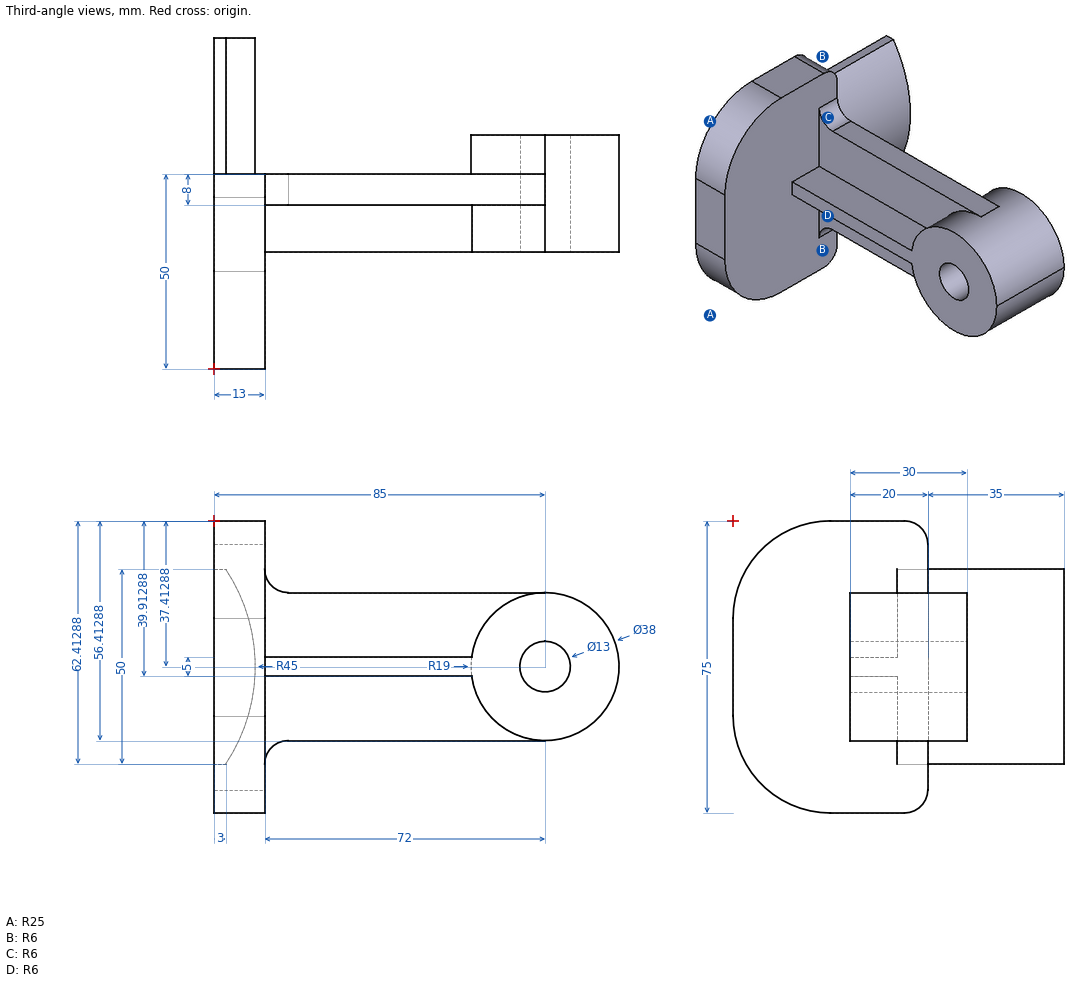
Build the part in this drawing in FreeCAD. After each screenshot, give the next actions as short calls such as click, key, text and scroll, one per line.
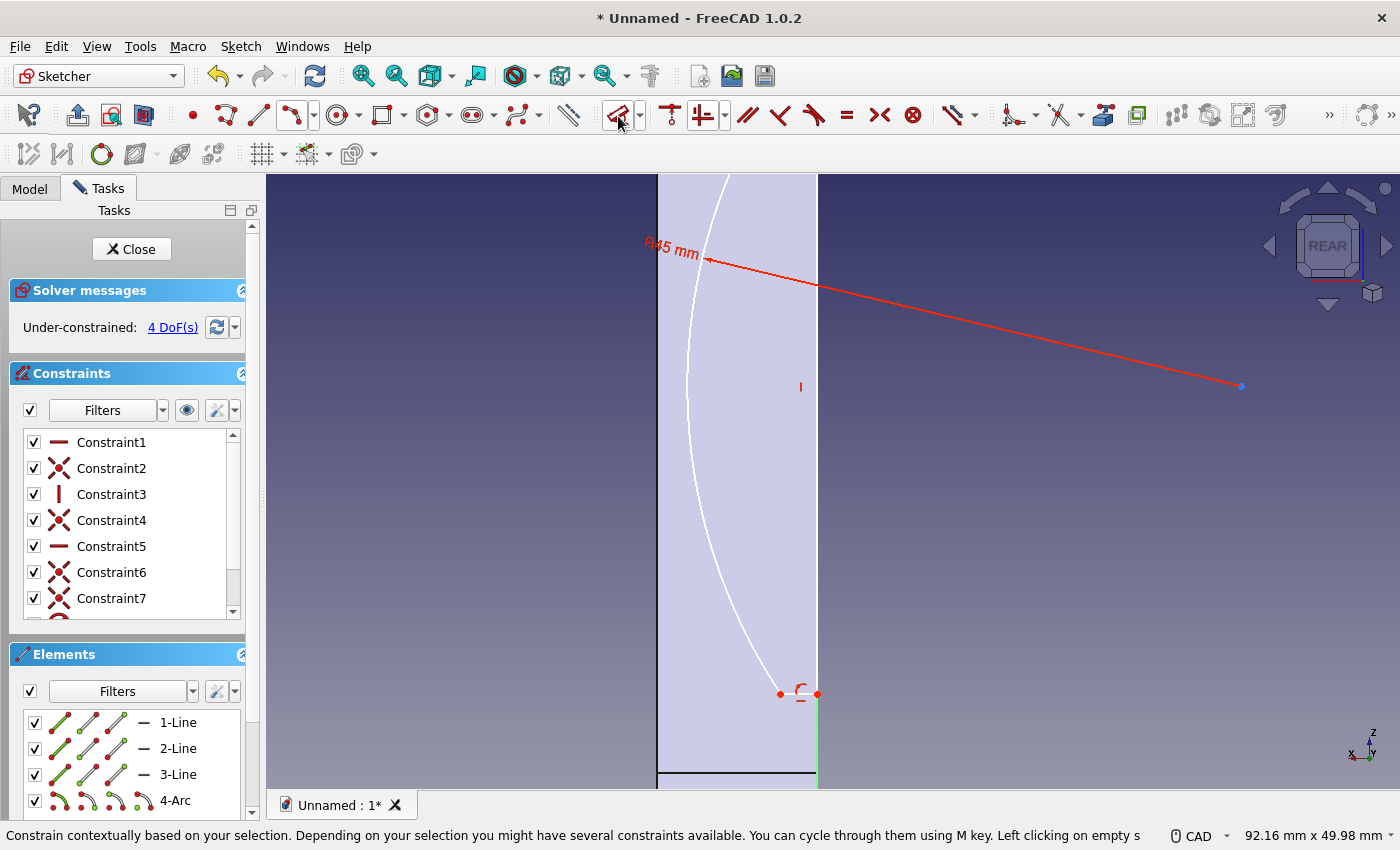
scroll(792, 694, up, 2)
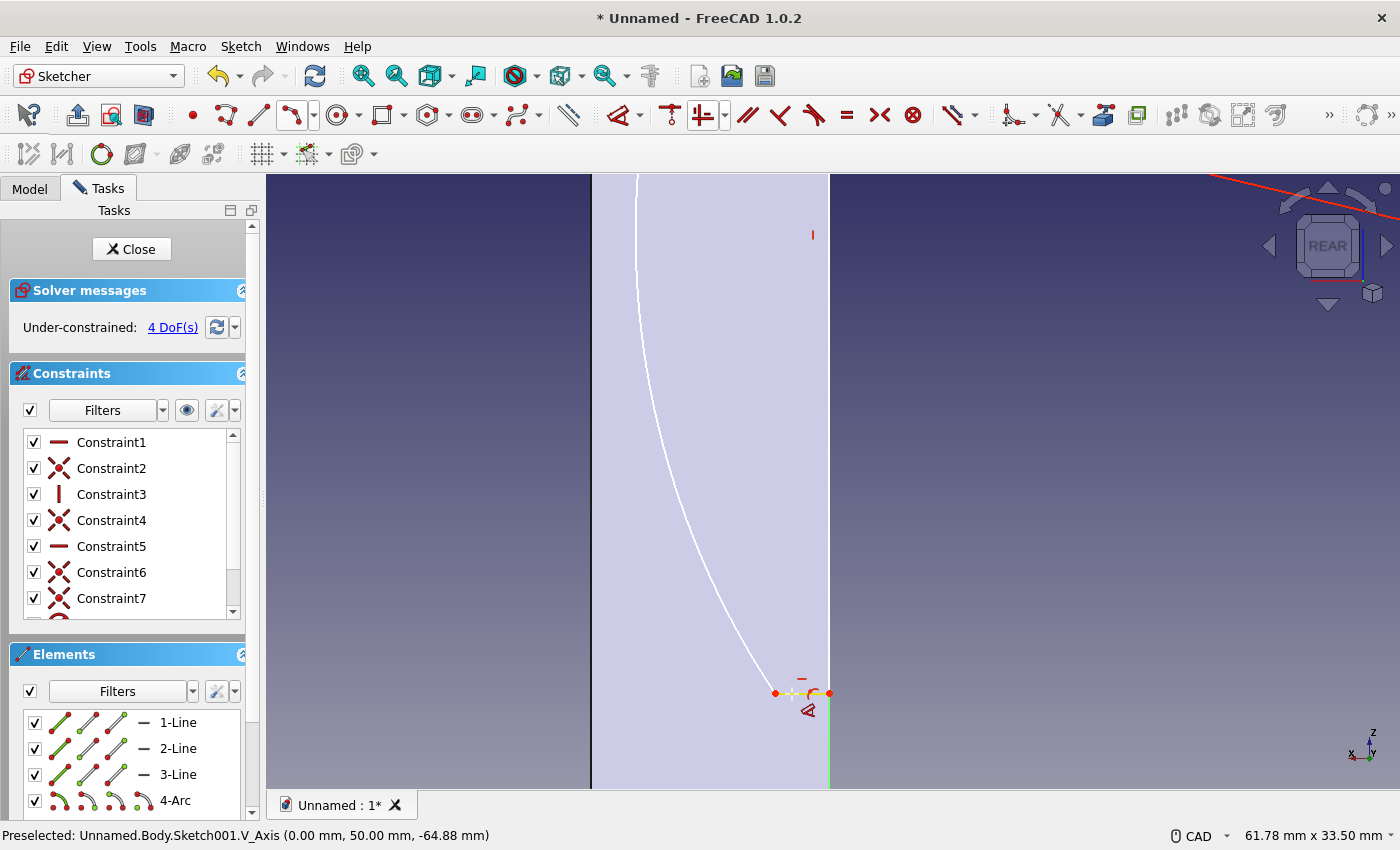
click(791, 694)
click(802, 728)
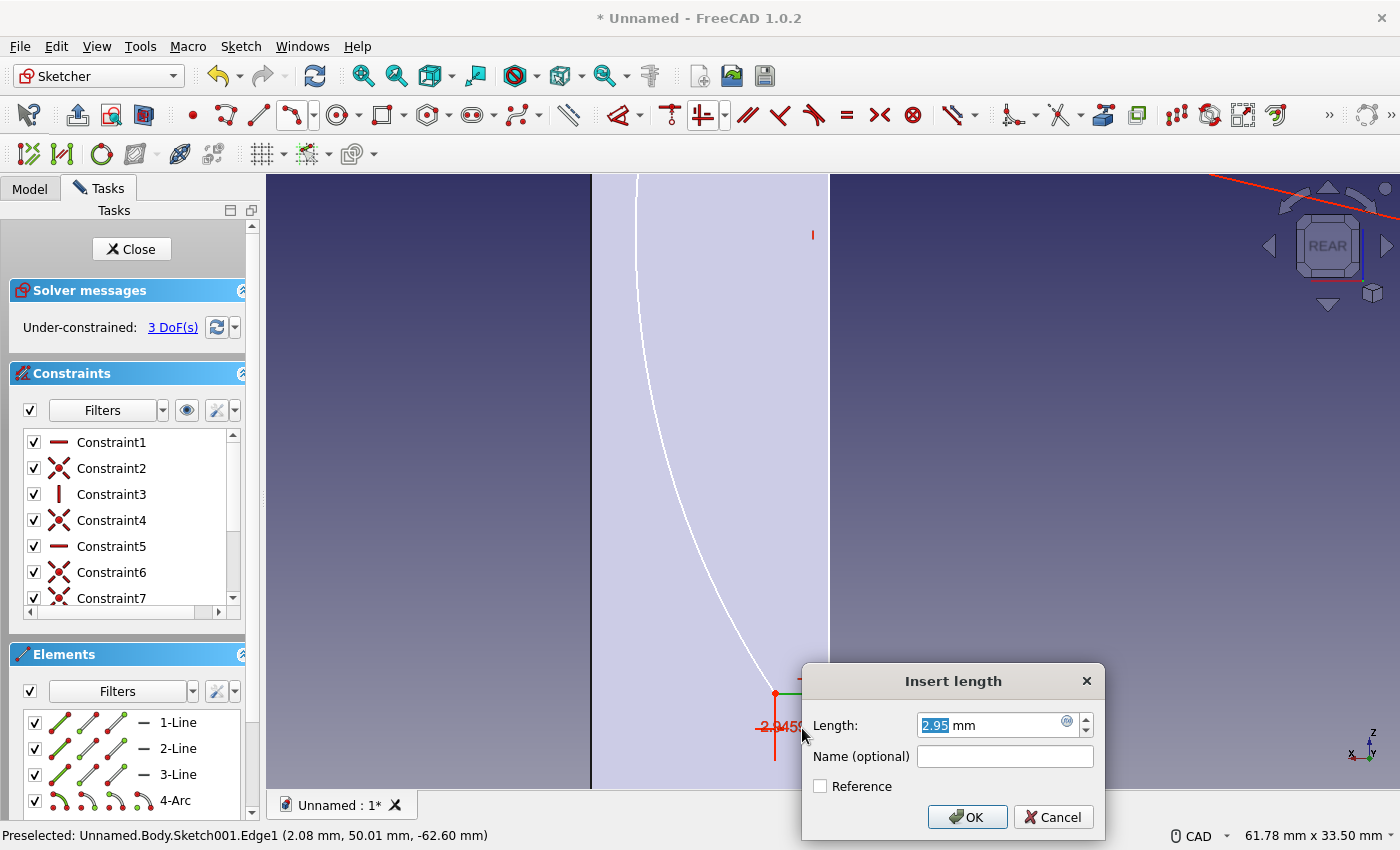
text(3)
key(Return)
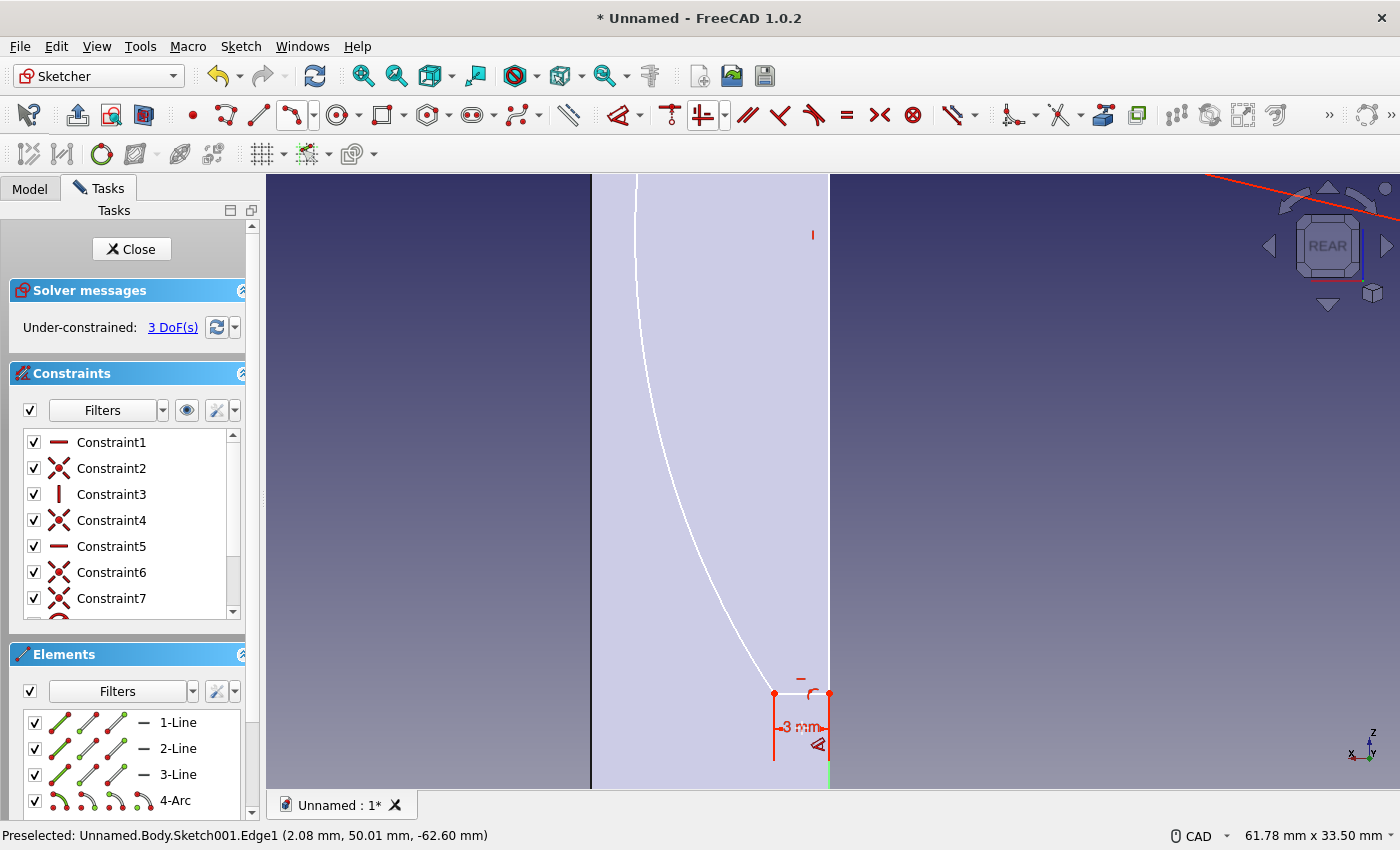
scroll(783, 693, down, 5)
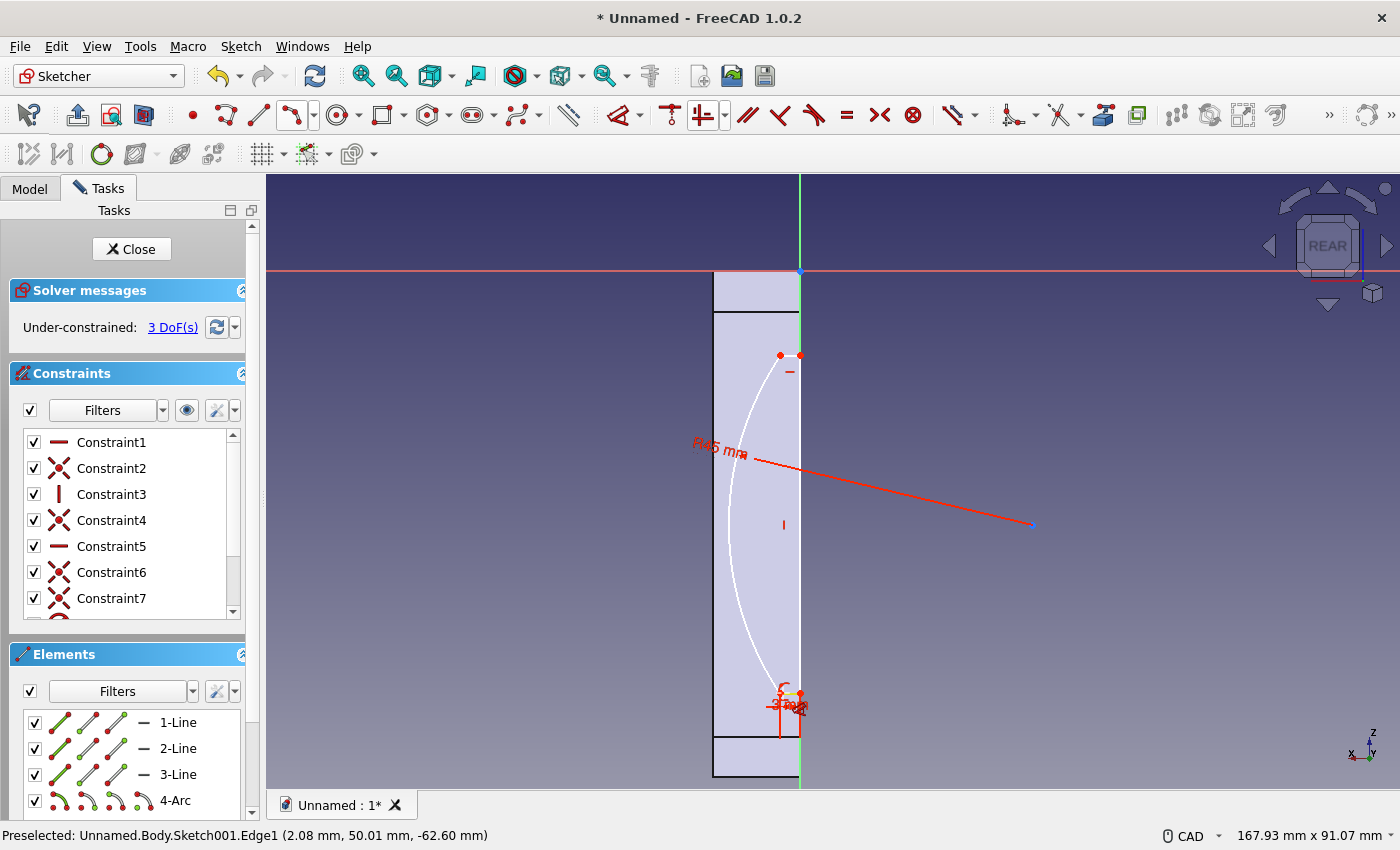
scroll(794, 356, up, 5)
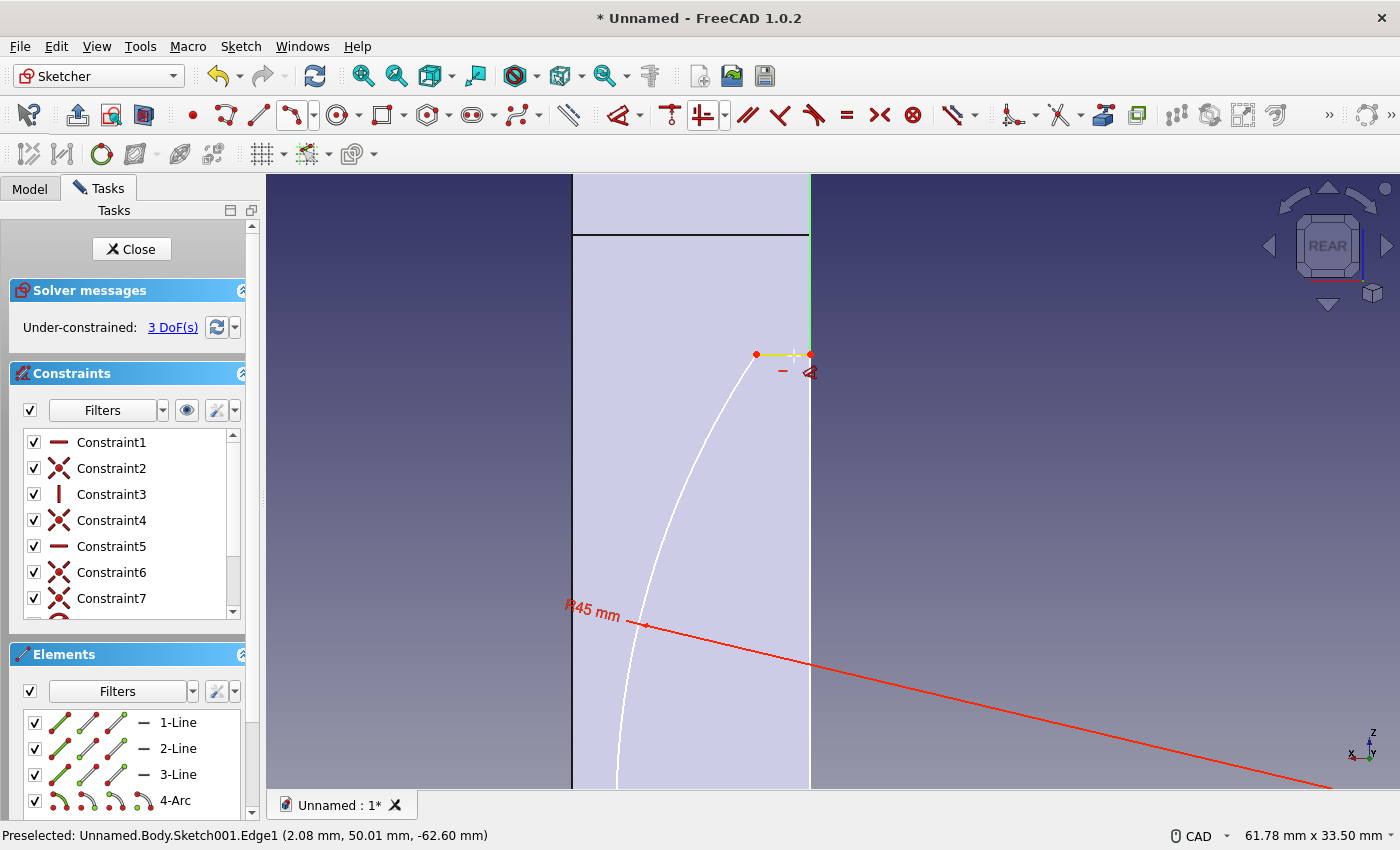
click(794, 355)
click(783, 321)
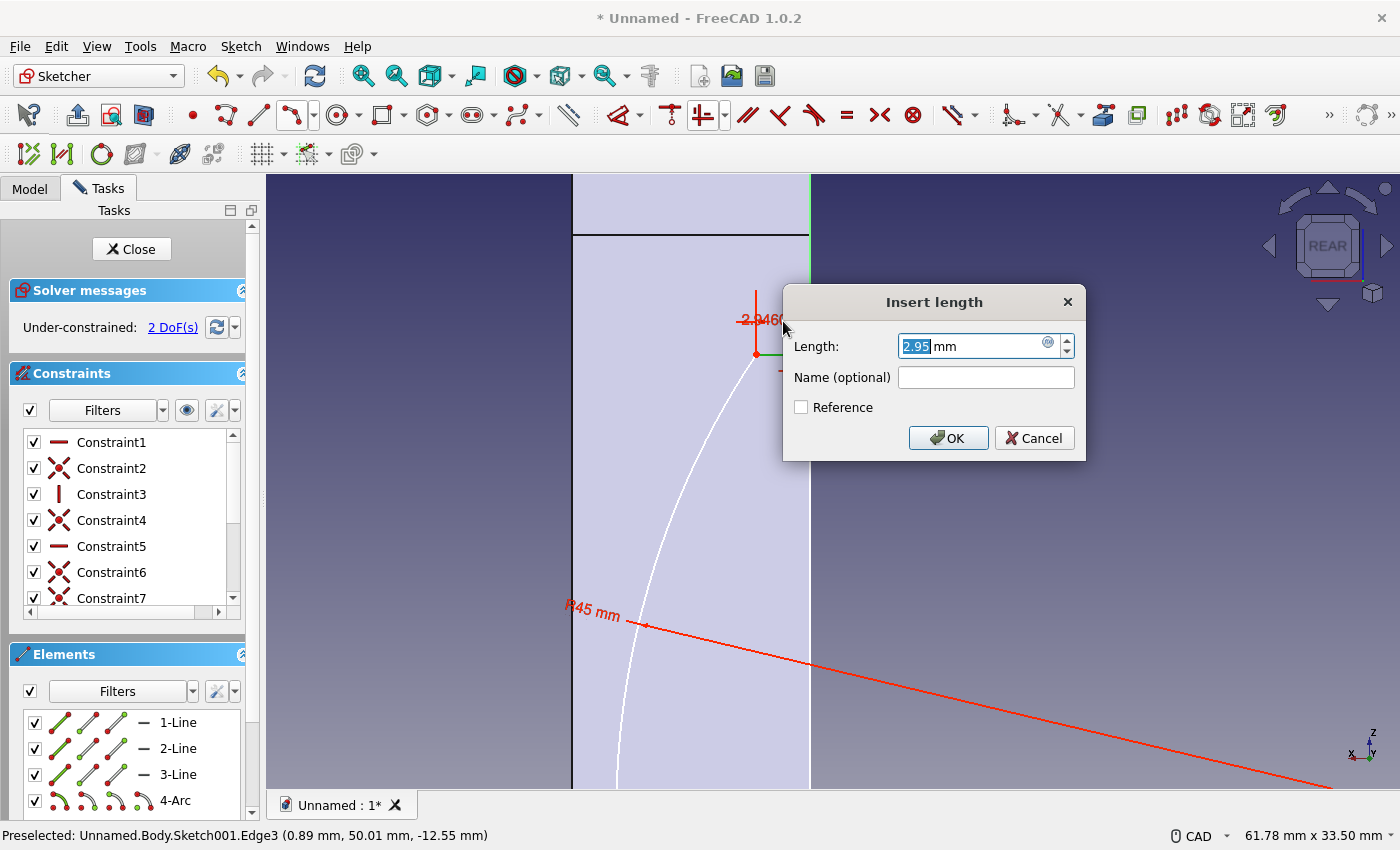
text(3)
key(Return)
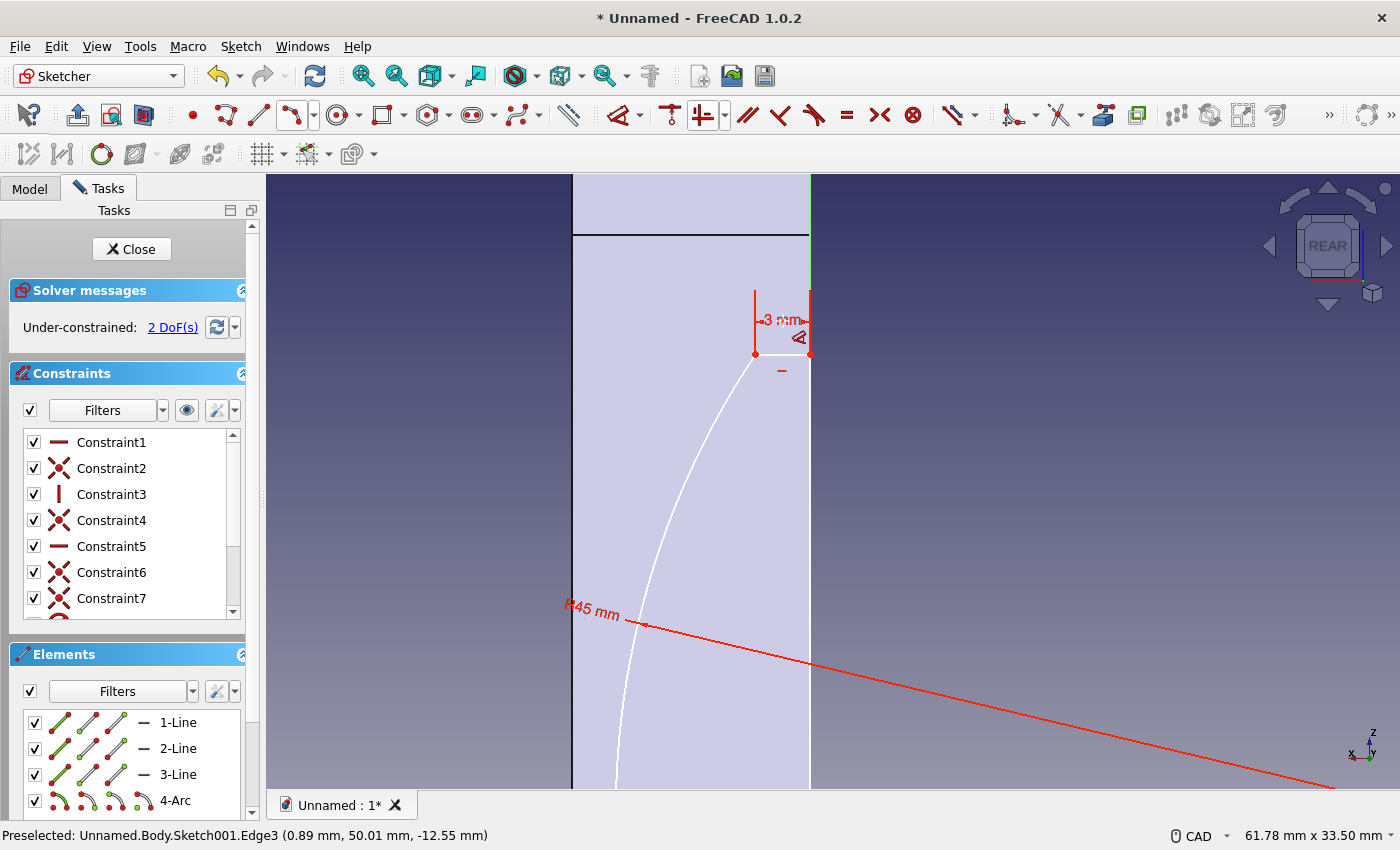
click(810, 630)
click(844, 558)